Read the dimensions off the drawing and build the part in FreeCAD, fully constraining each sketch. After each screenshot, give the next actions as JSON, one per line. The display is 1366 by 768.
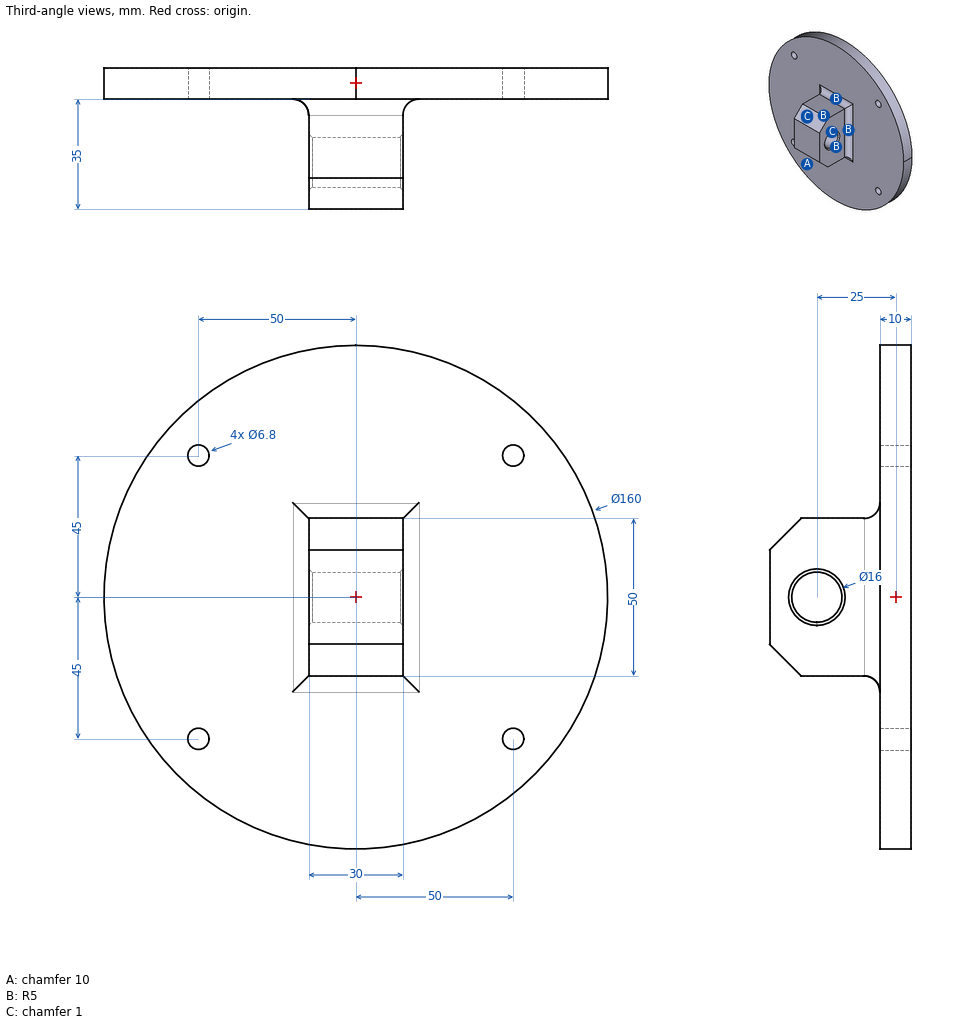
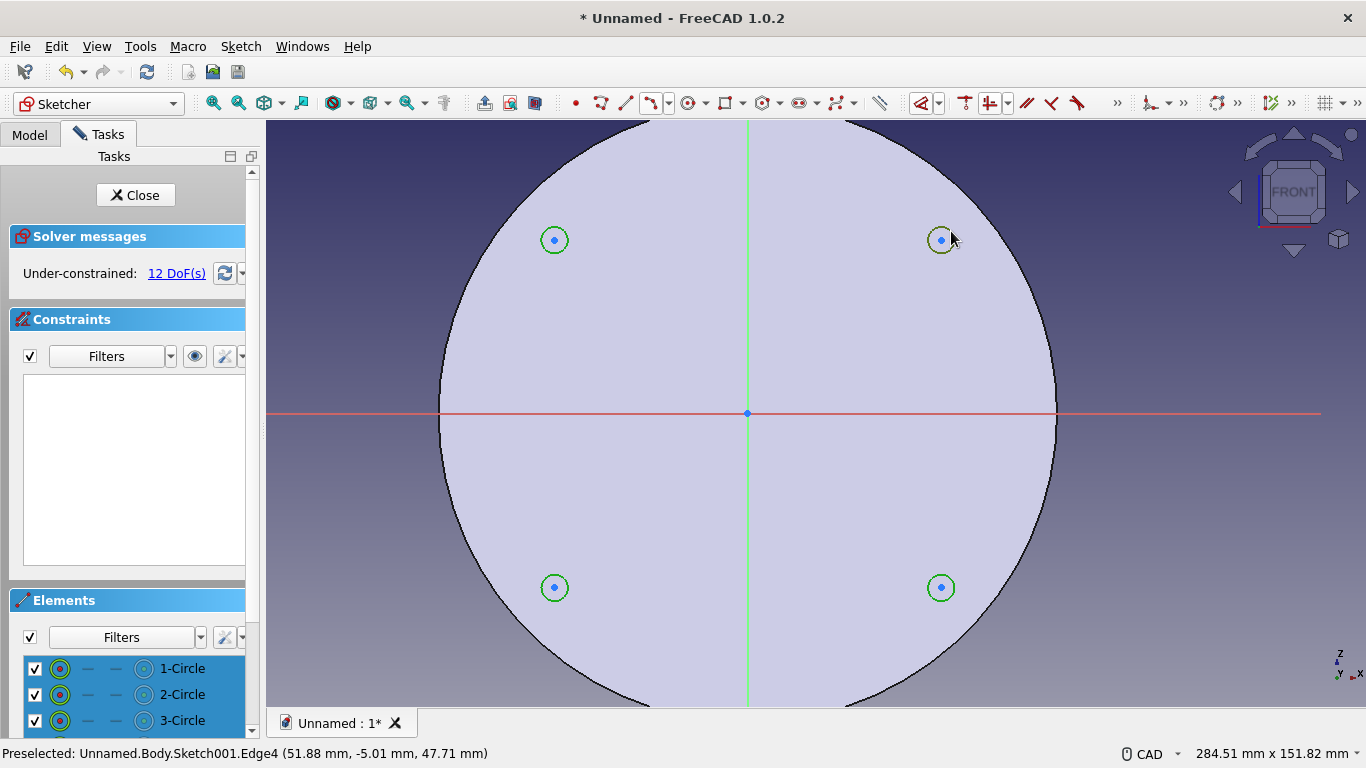
{"action": "key", "text": "e"}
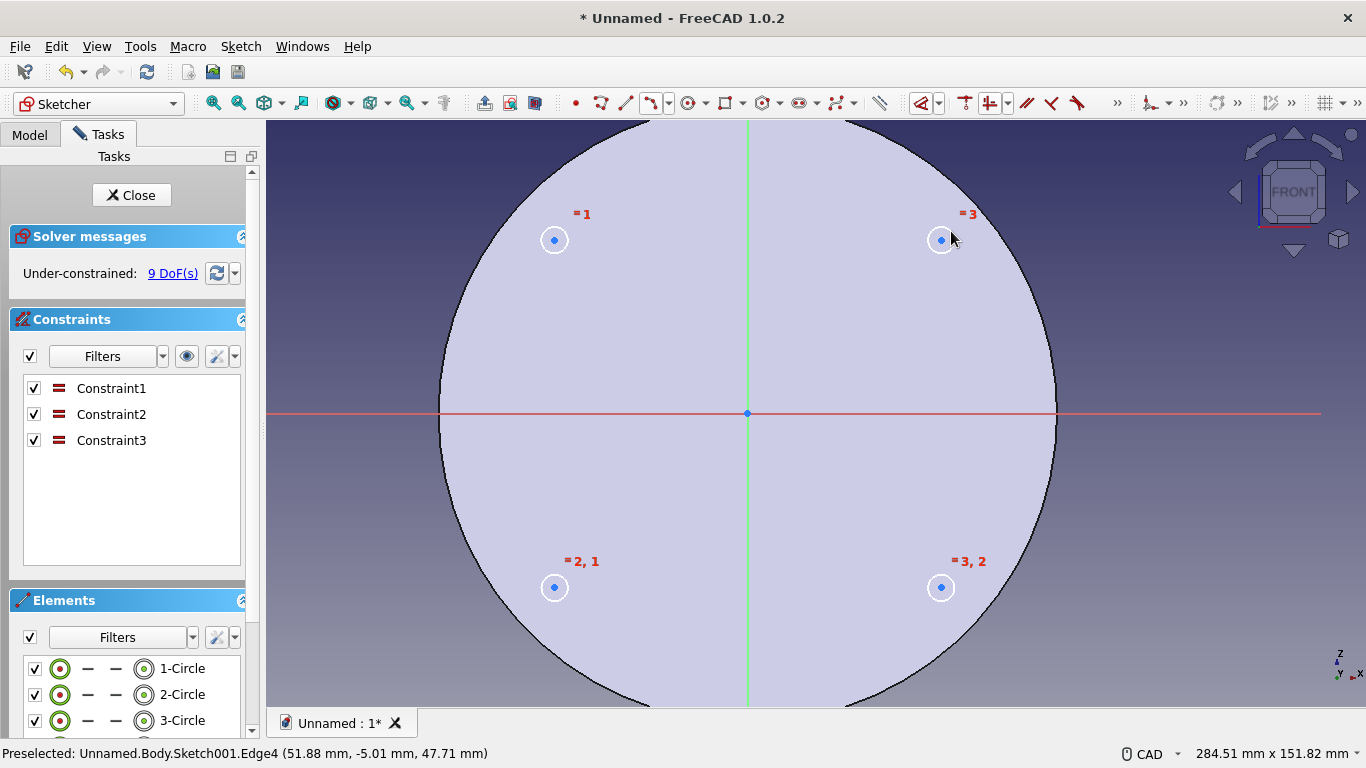
{"action": "left_click", "coordinate": [555, 240]}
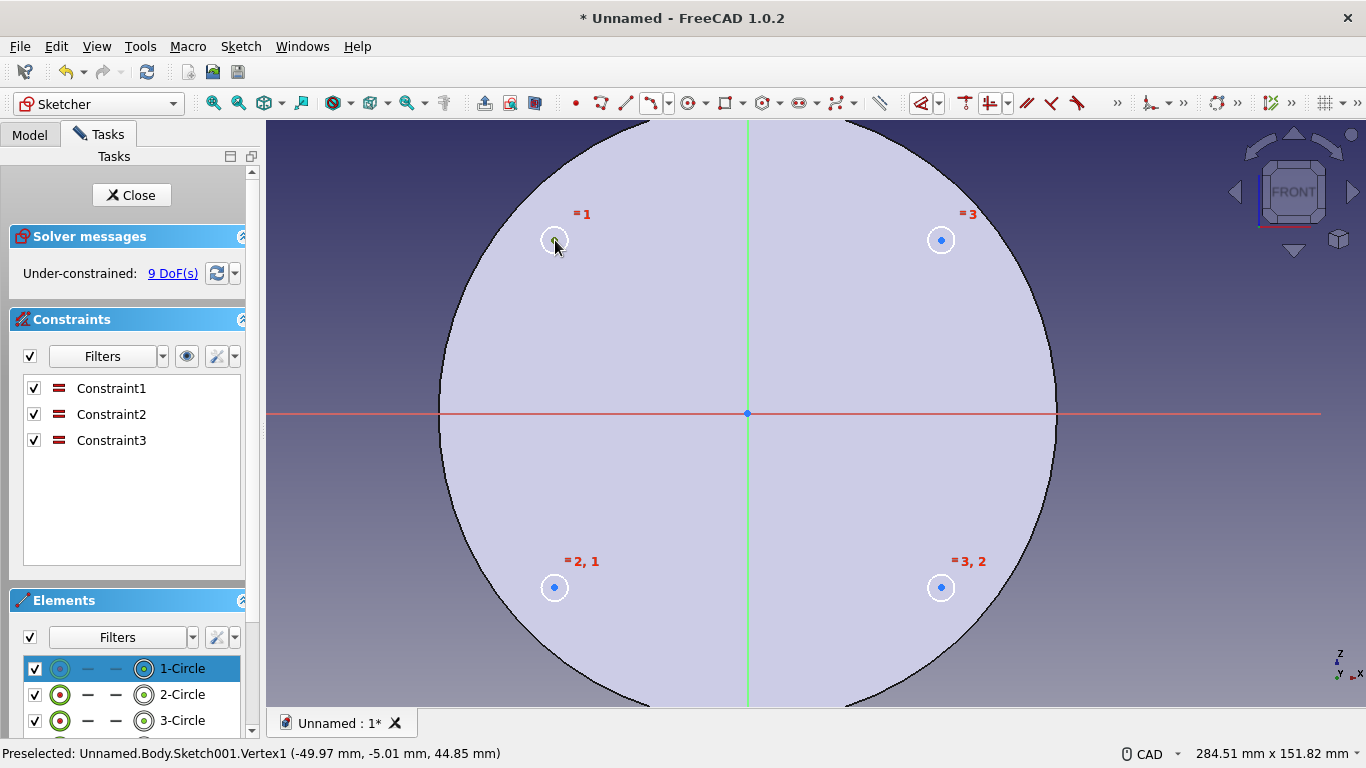
{"action": "left_click", "coordinate": [555, 588]}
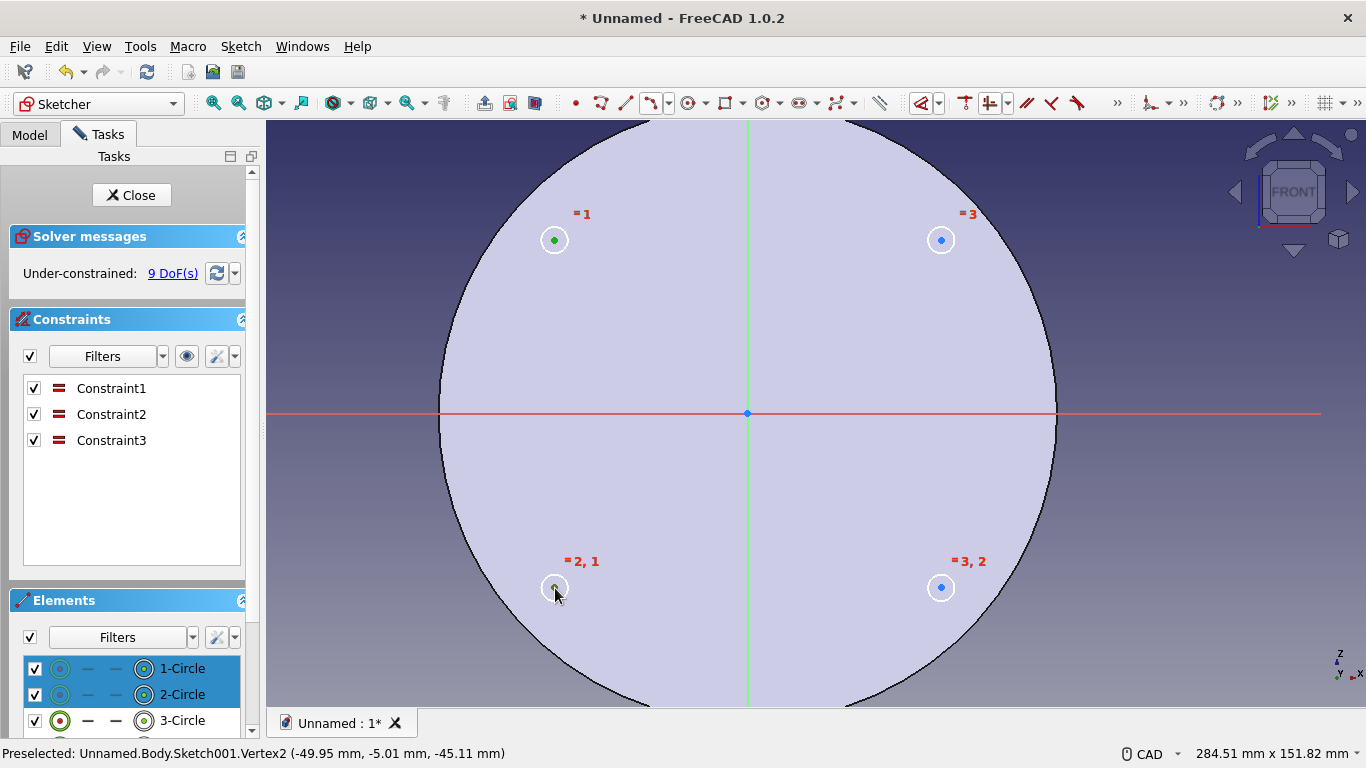
{"action": "key", "text": "v"}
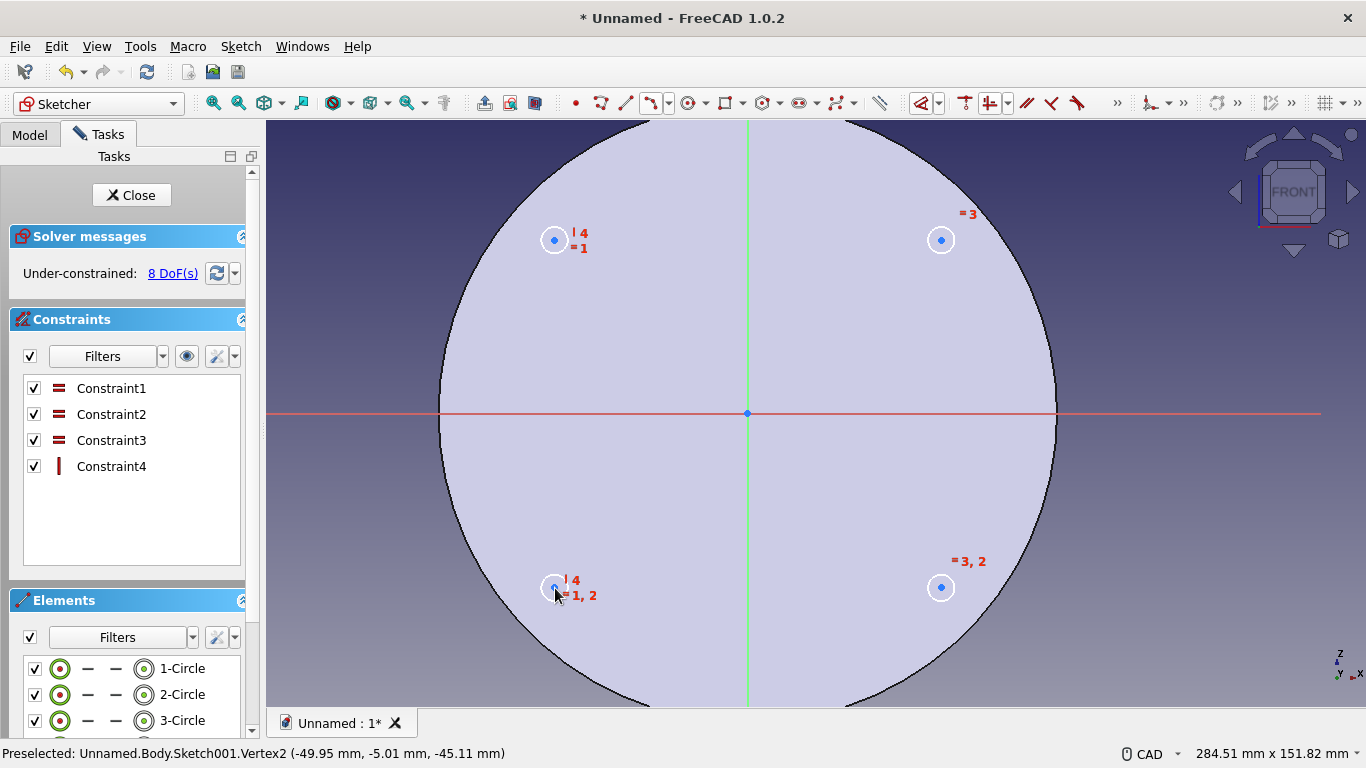
{"action": "left_click", "coordinate": [555, 588]}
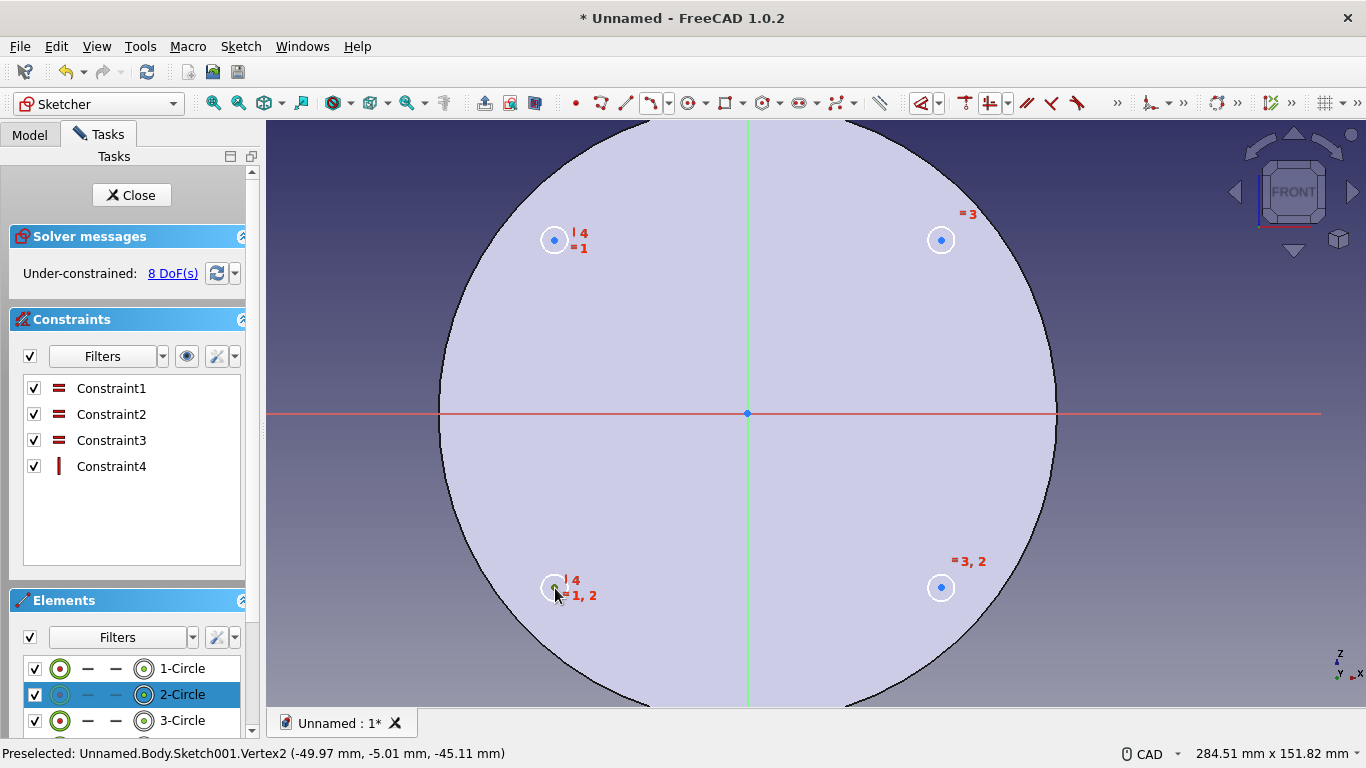
{"action": "left_click", "coordinate": [941, 588]}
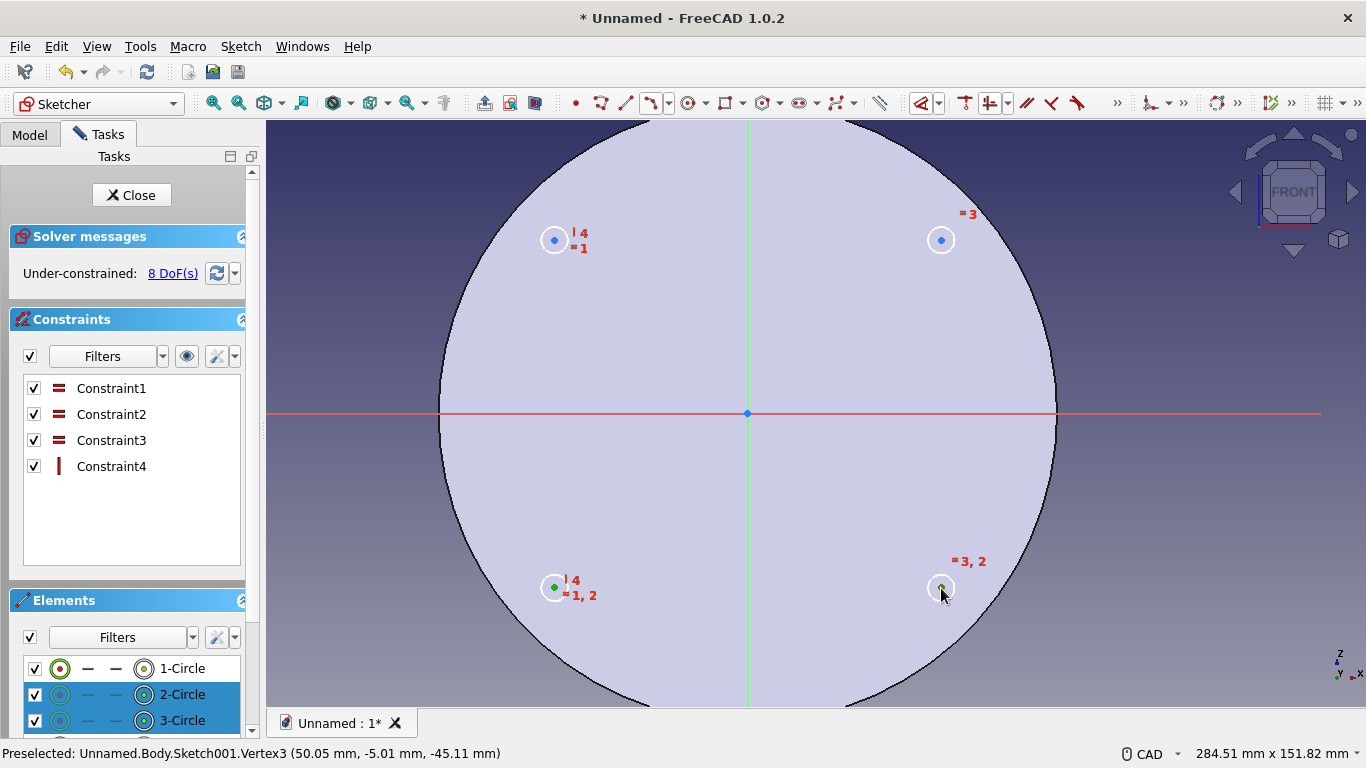
{"action": "key", "text": "h"}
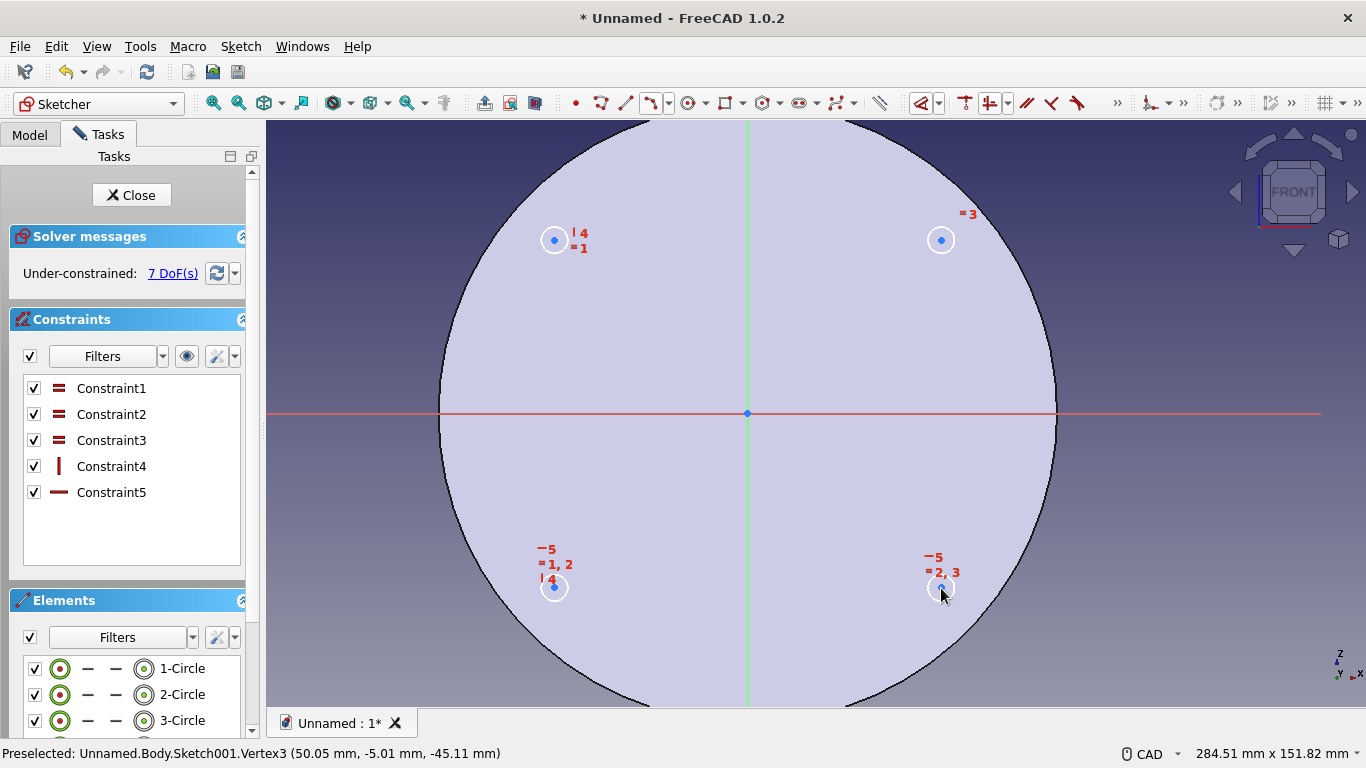
{"action": "left_click", "coordinate": [941, 588]}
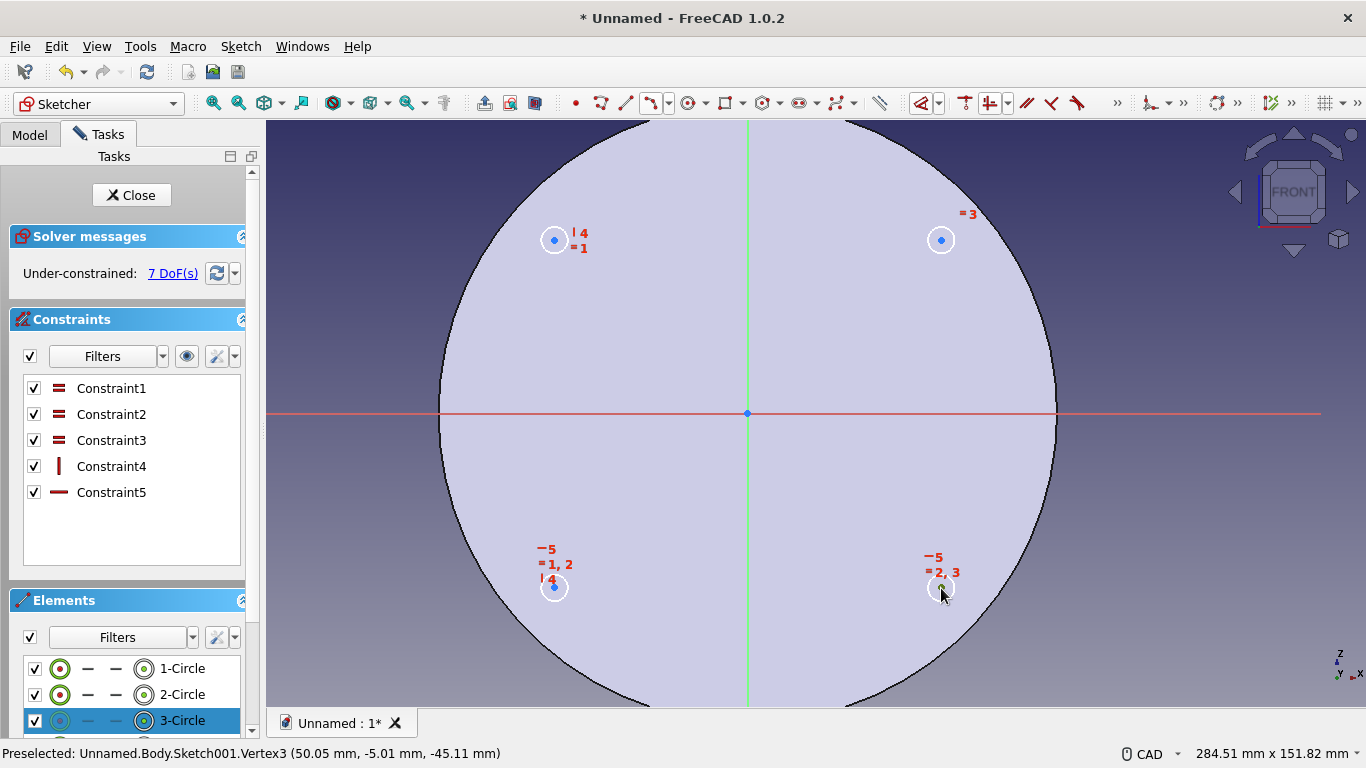
{"action": "left_click", "coordinate": [941, 240]}